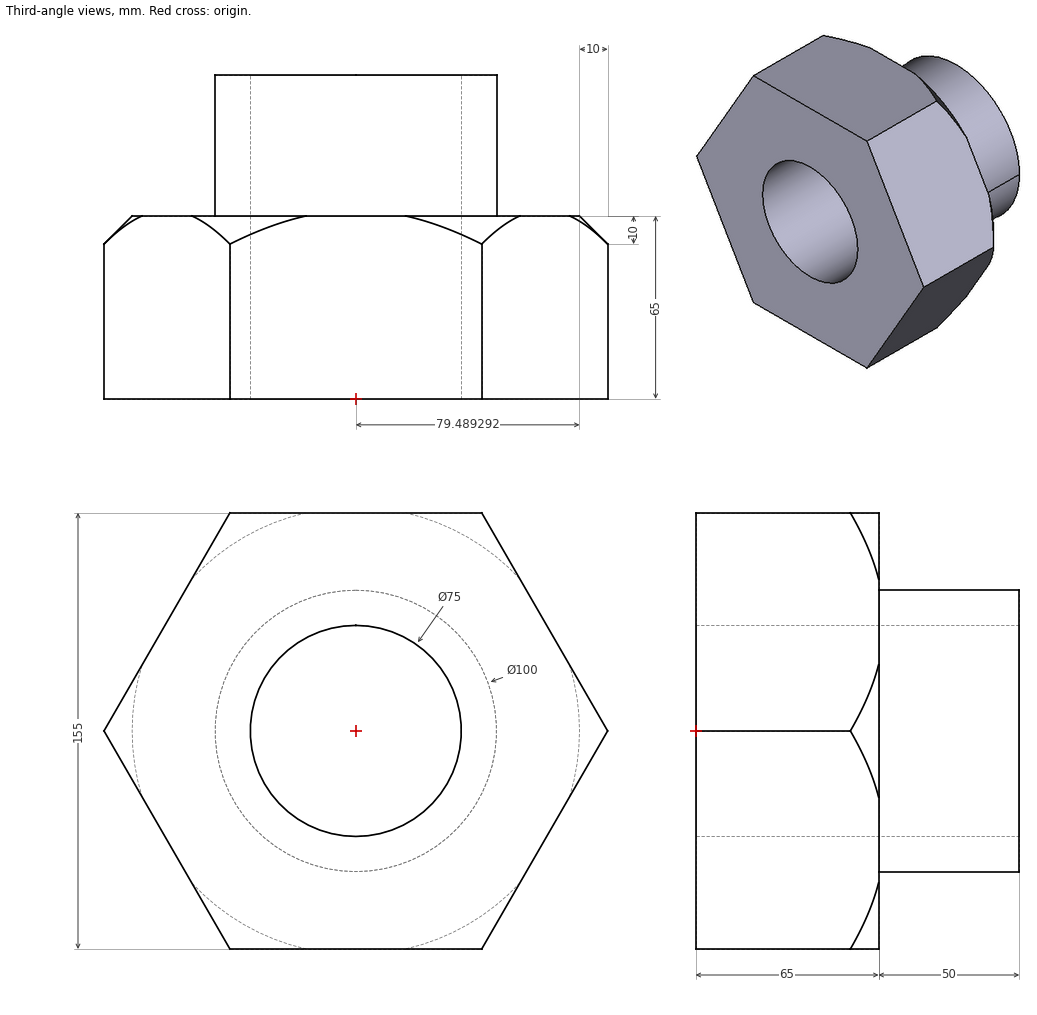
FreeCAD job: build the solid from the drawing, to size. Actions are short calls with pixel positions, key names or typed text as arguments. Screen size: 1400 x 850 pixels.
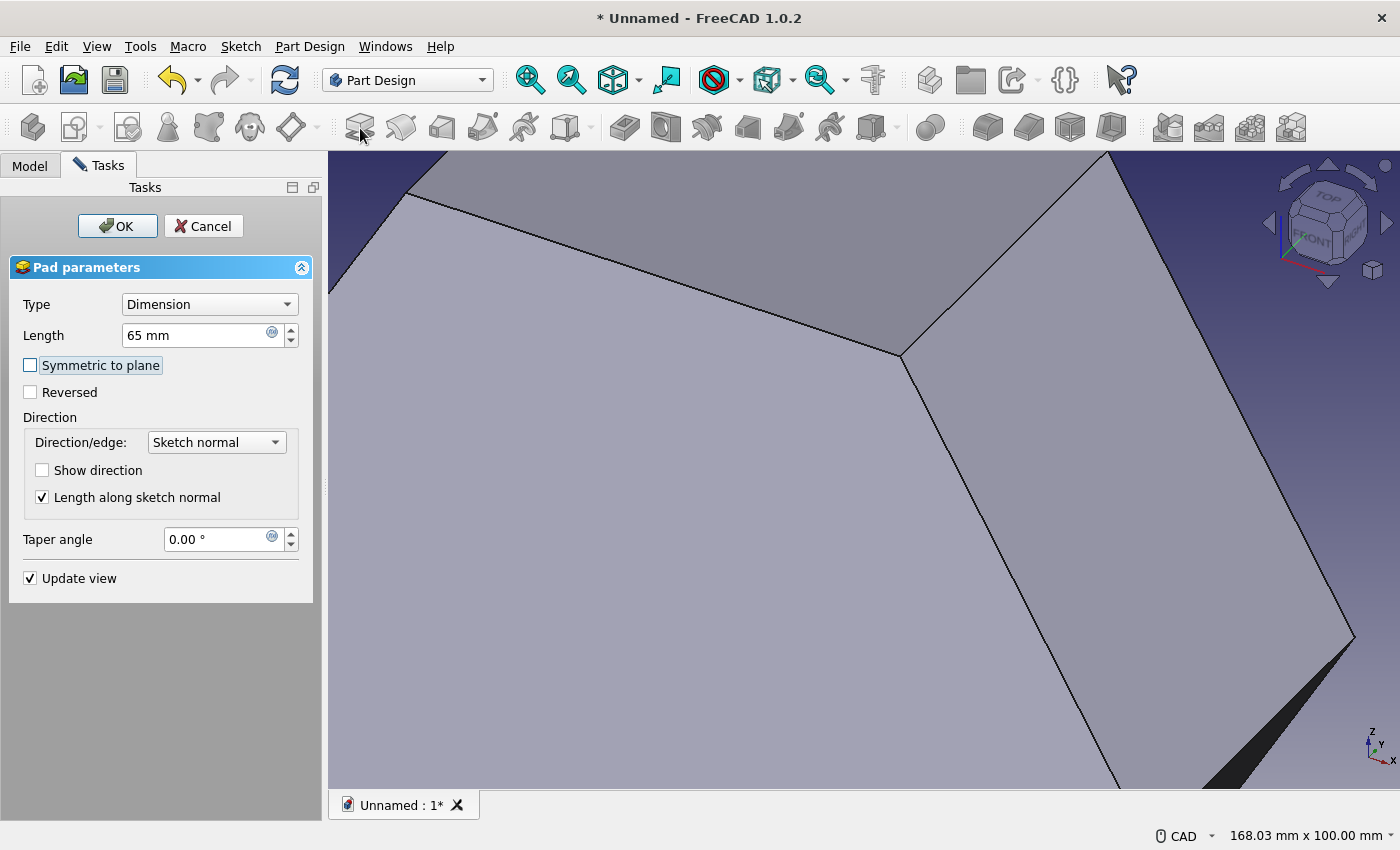
click(31, 392)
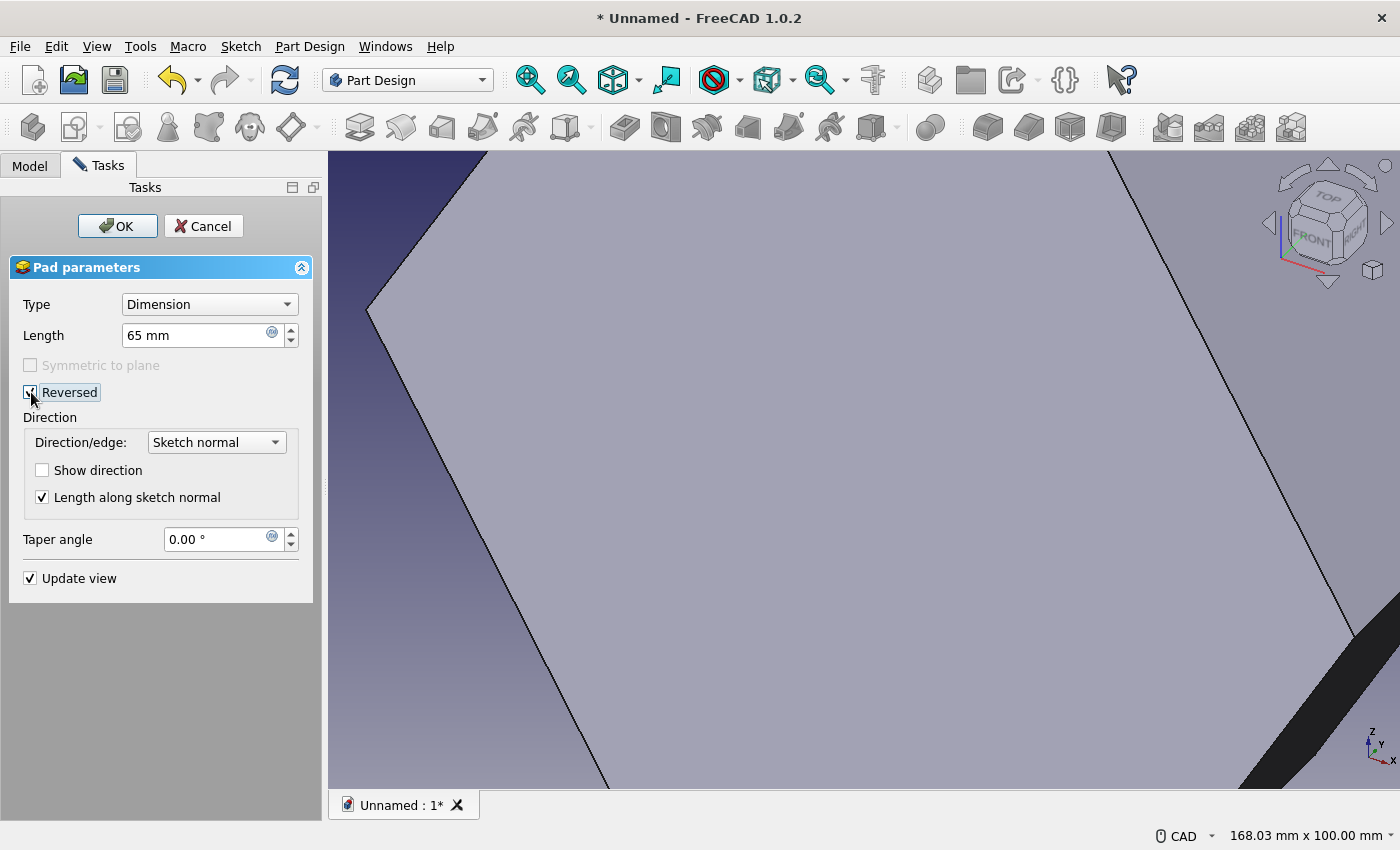
click(118, 226)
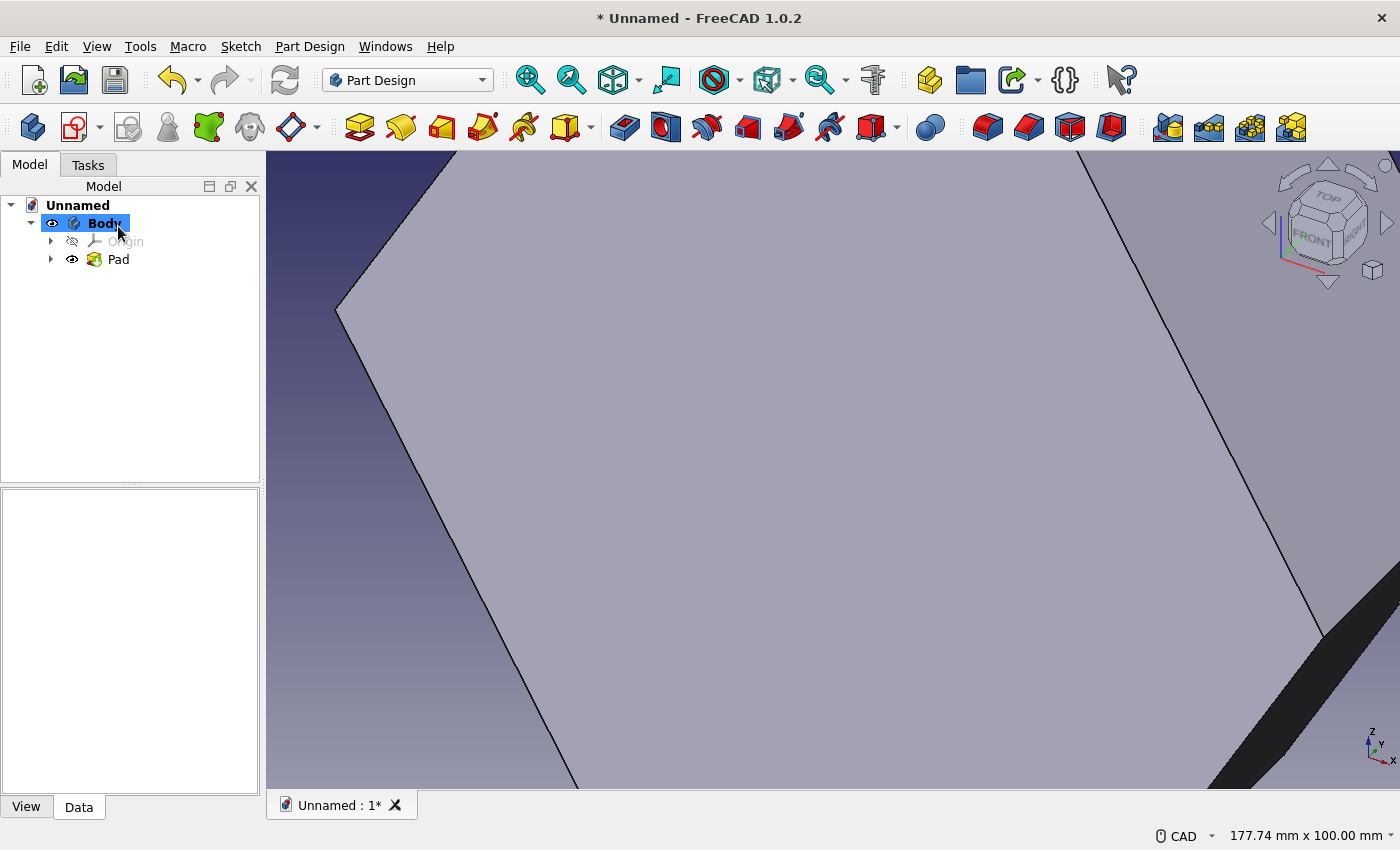
click(531, 80)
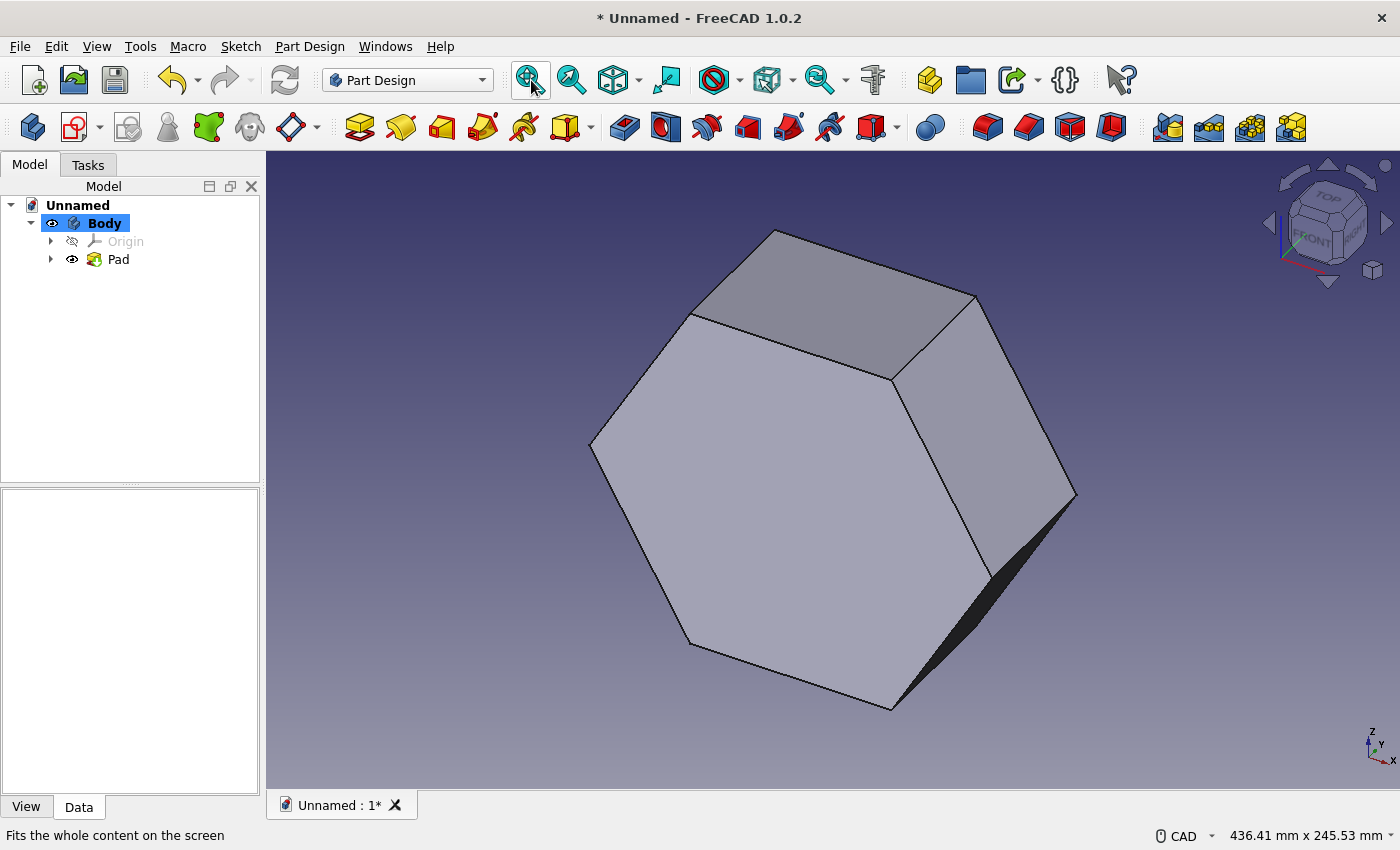
click(74, 128)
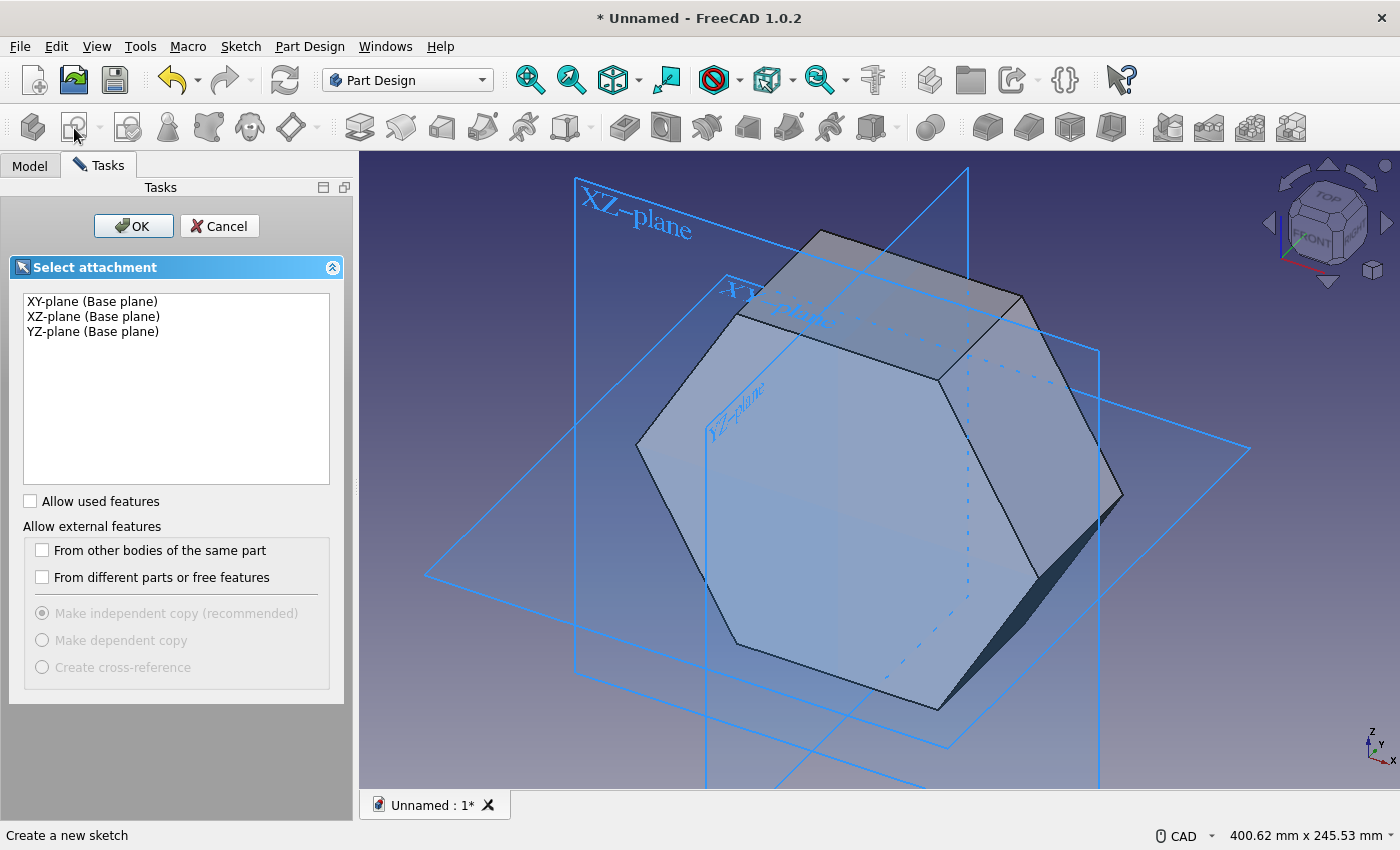
click(84, 302)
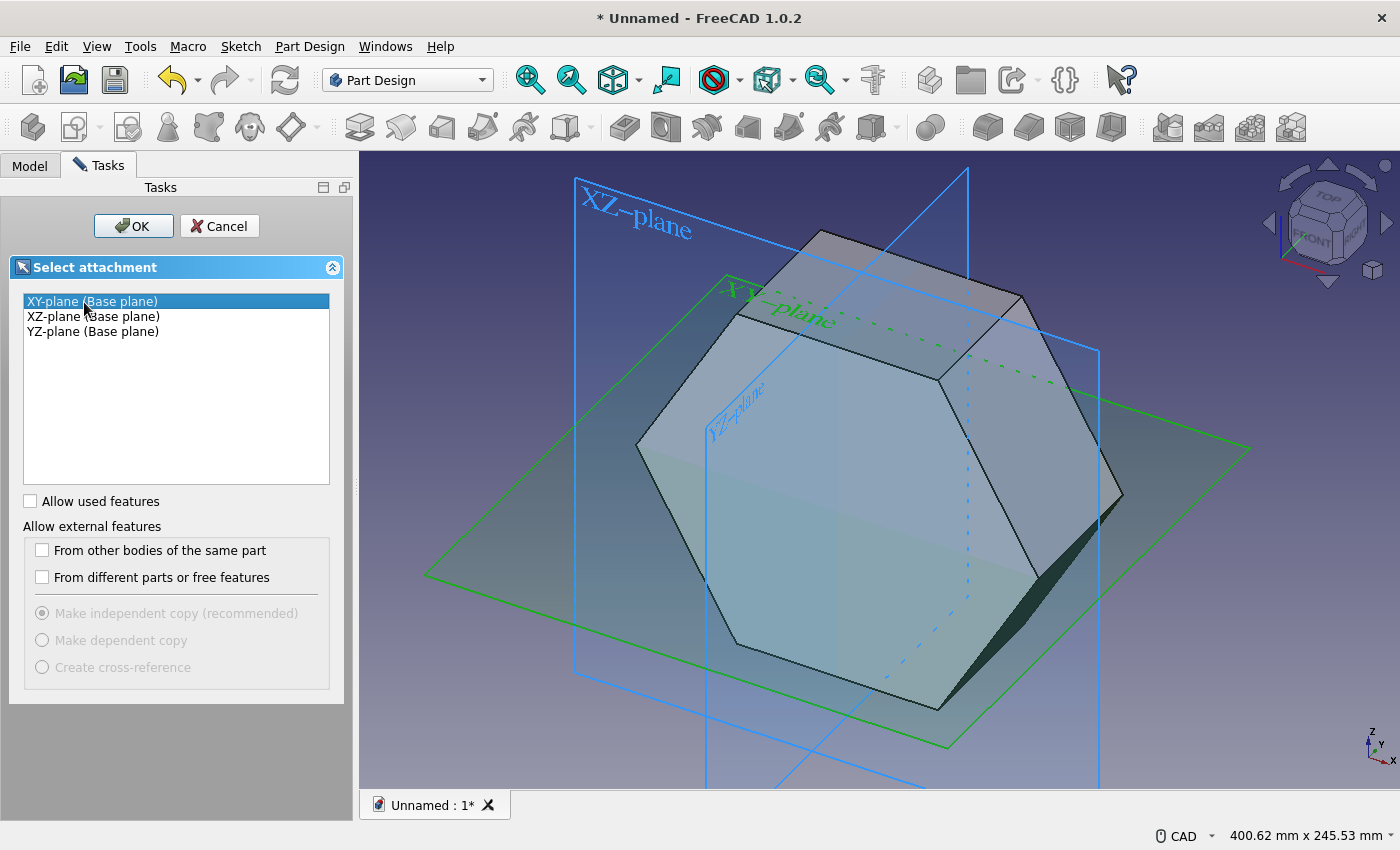
click(134, 226)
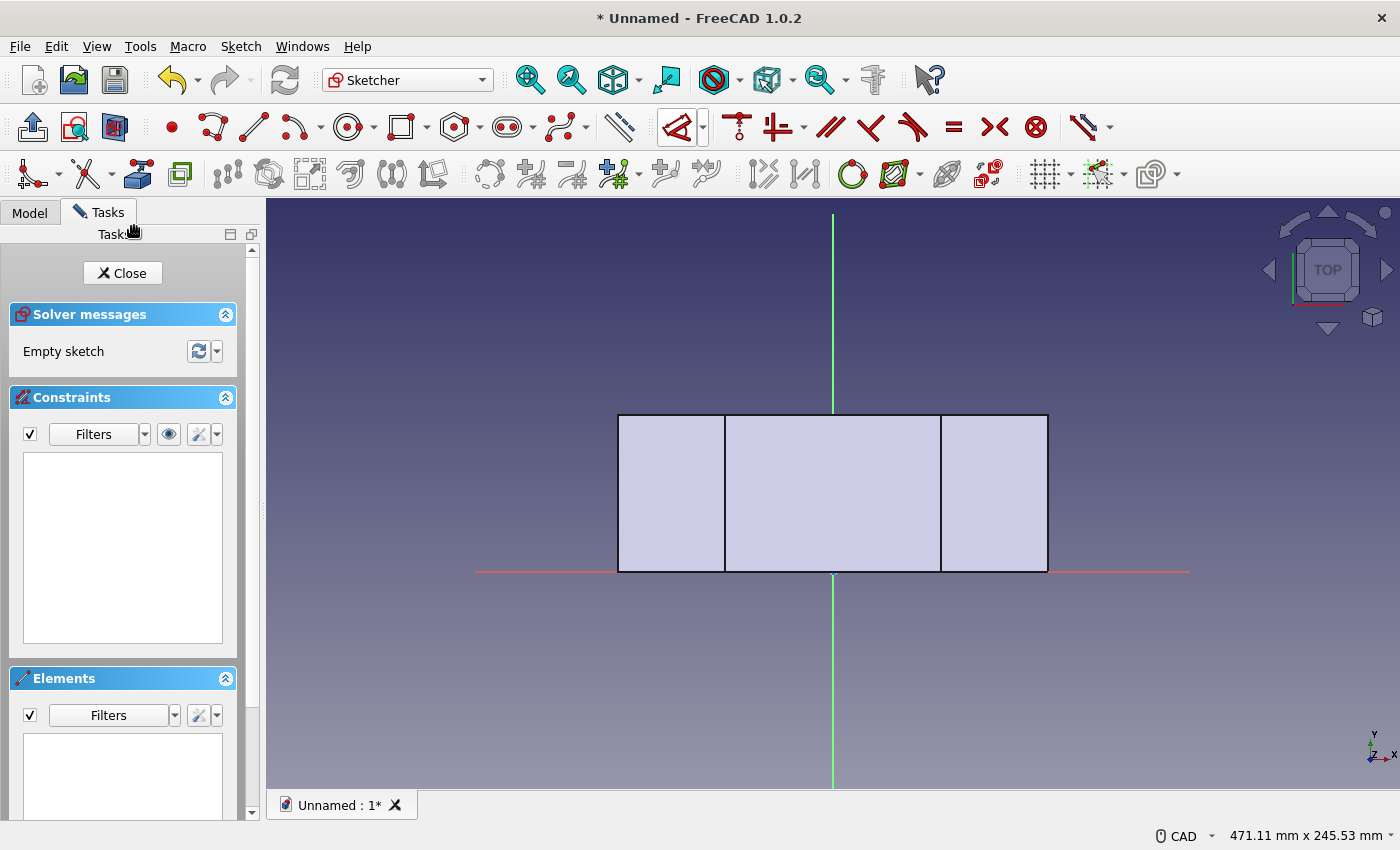
click(115, 128)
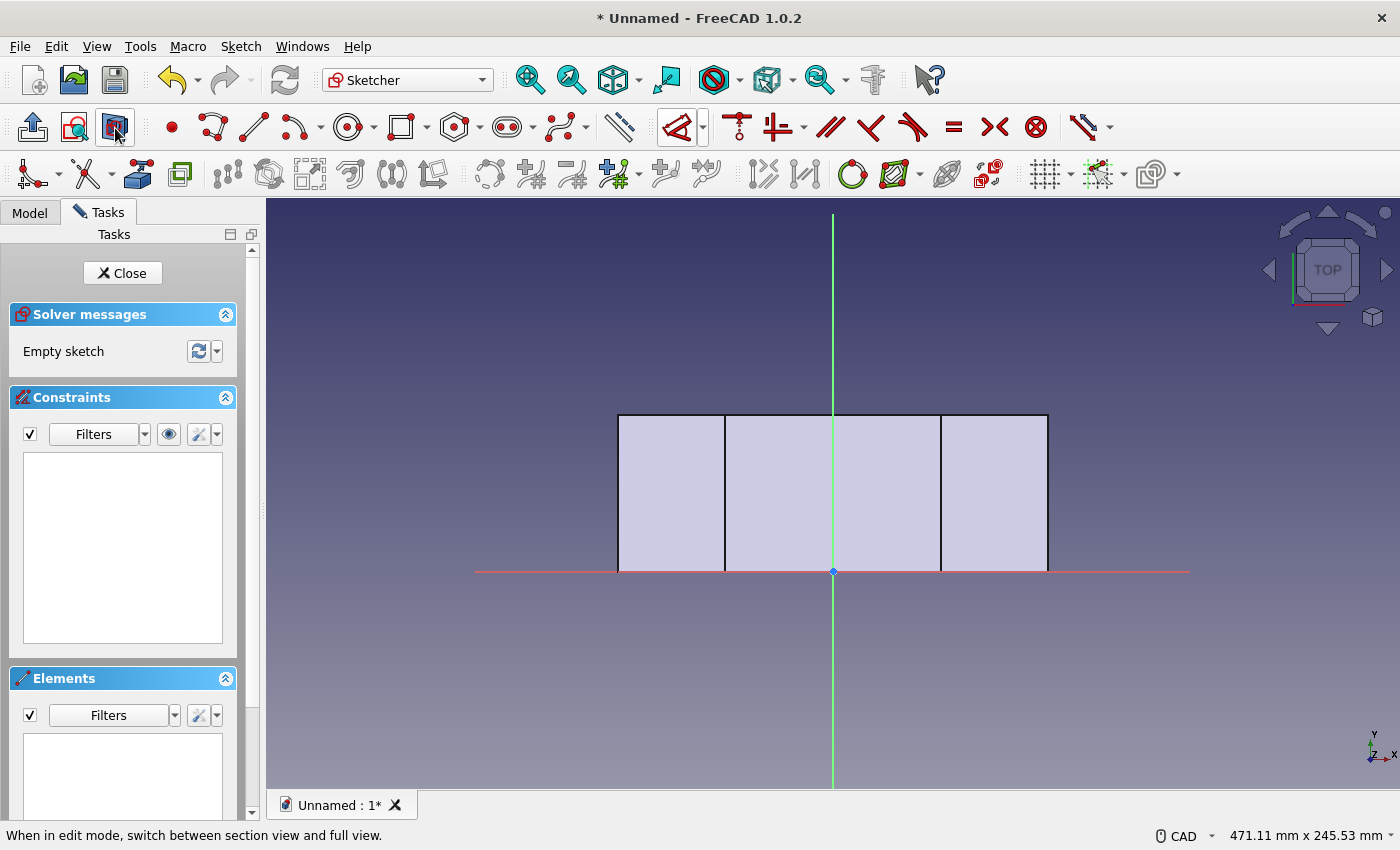
scroll(1054, 423, up, 14)